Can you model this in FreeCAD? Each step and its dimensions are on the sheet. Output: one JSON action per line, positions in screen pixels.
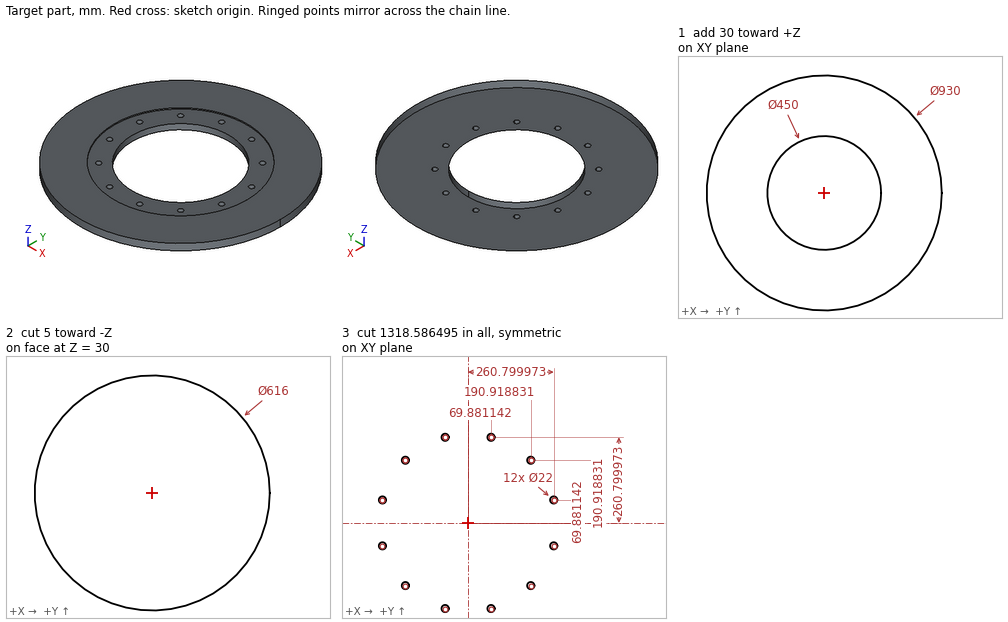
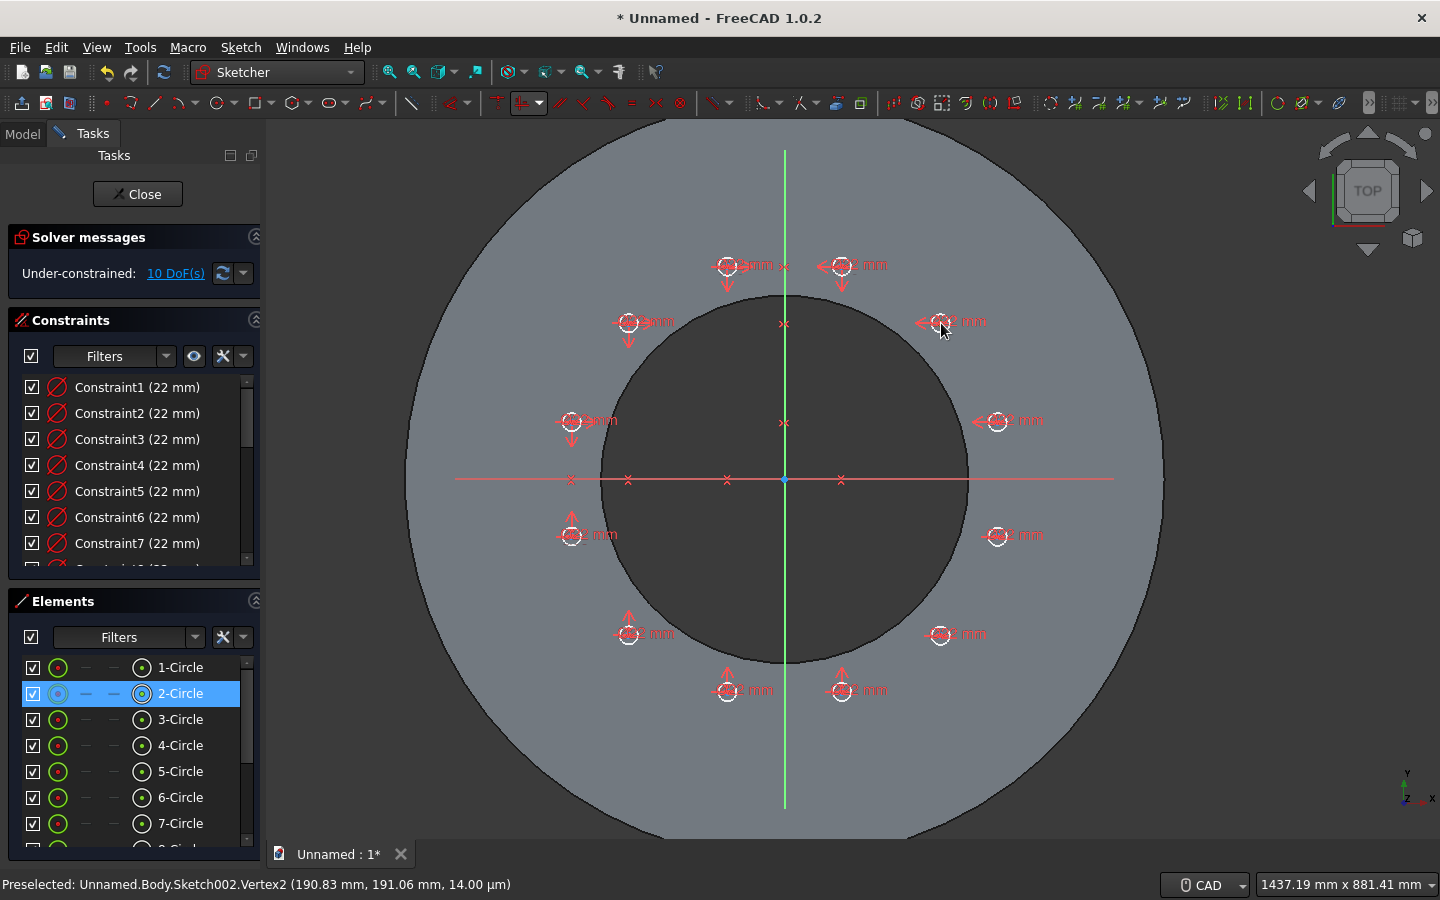
{"action": "left_click", "coordinate": [941, 636]}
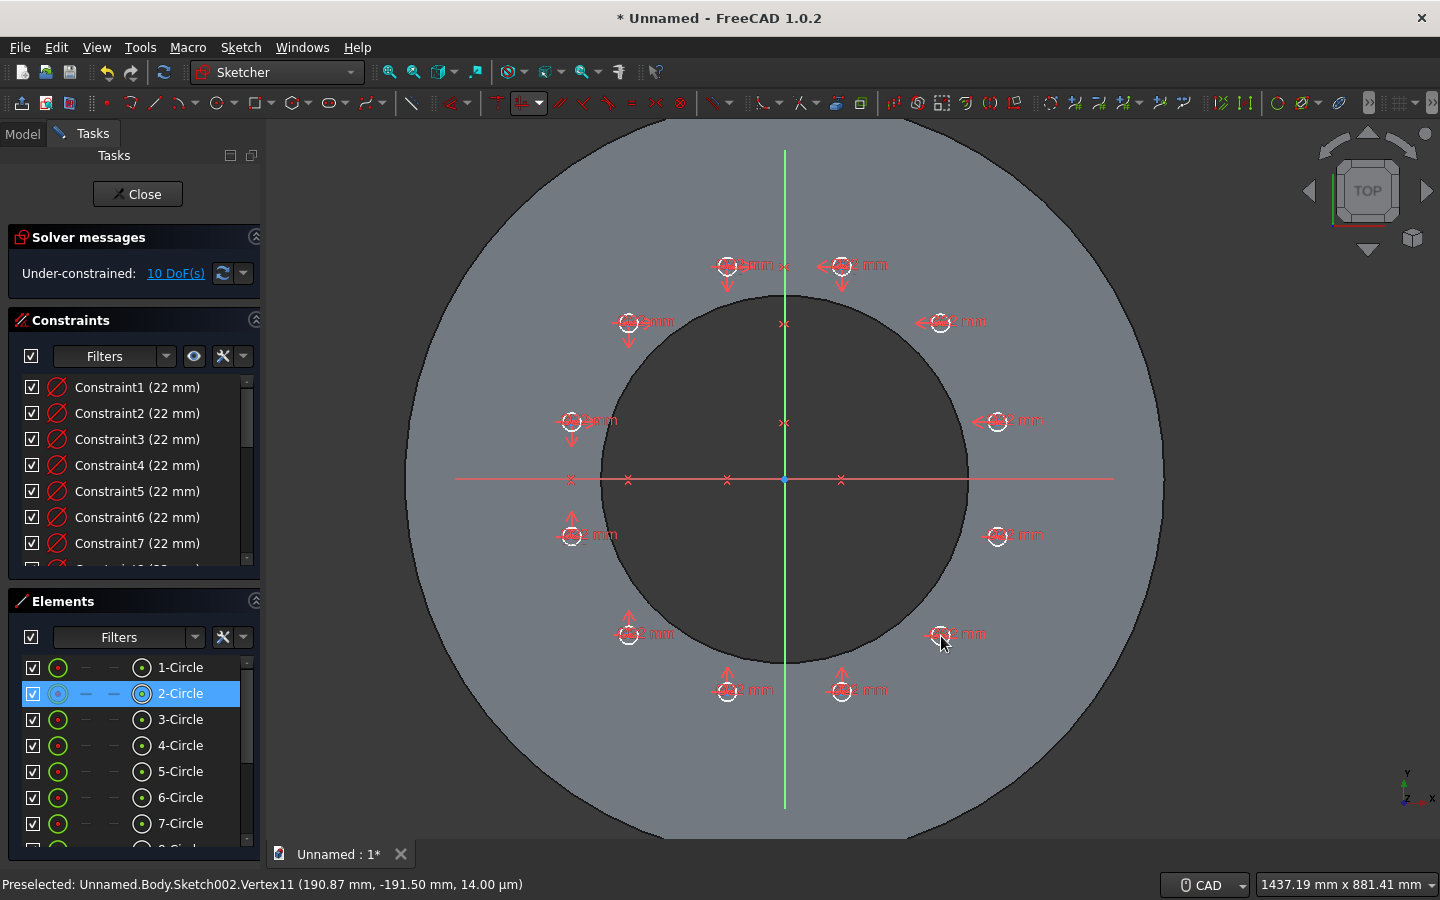
{"action": "left_click", "coordinate": [504, 479]}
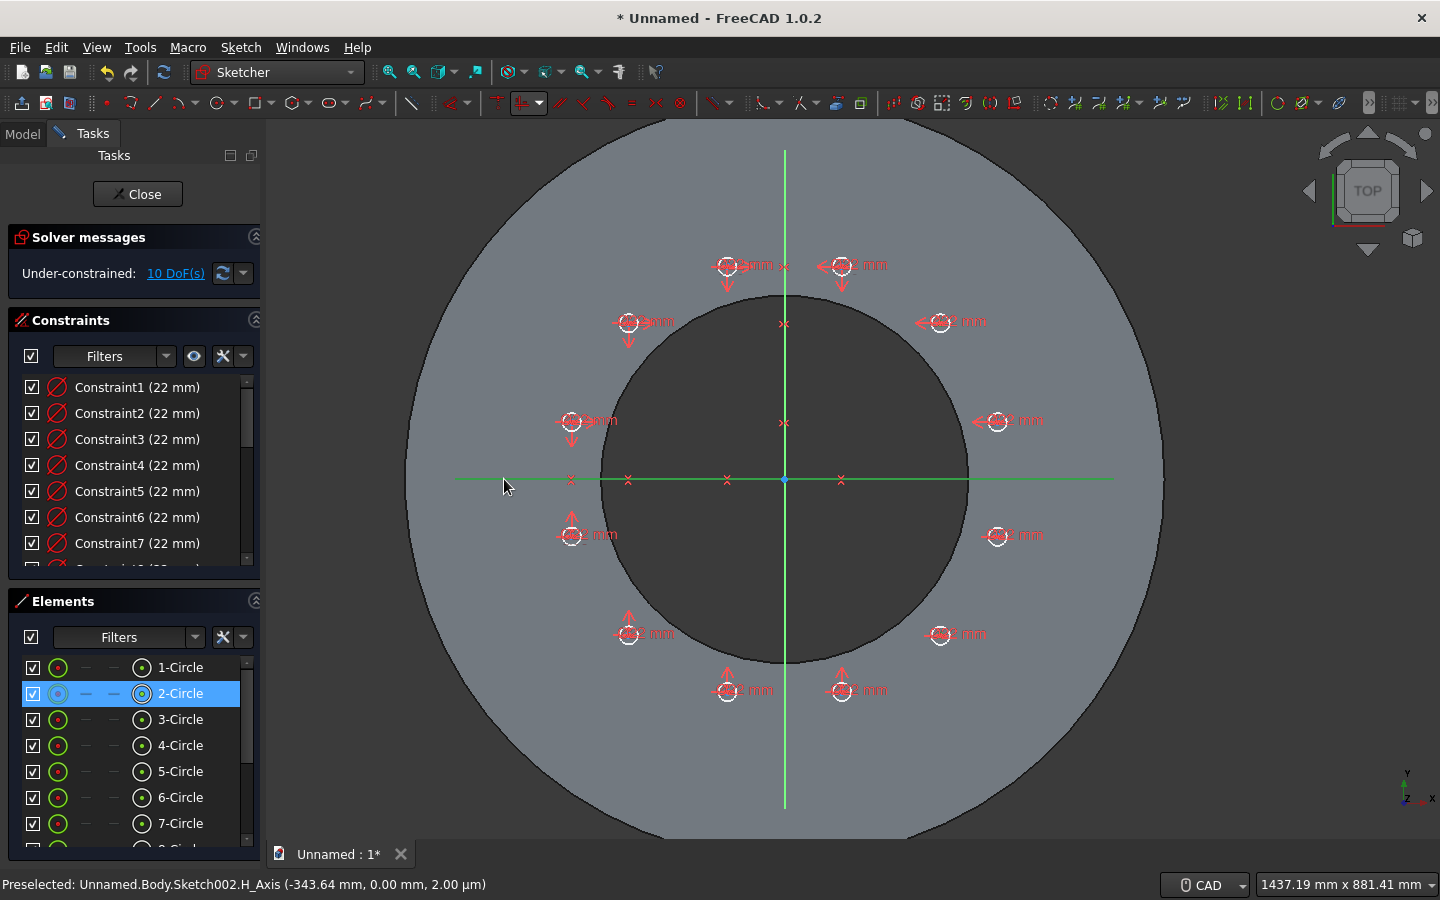
{"action": "left_click", "coordinate": [656, 104]}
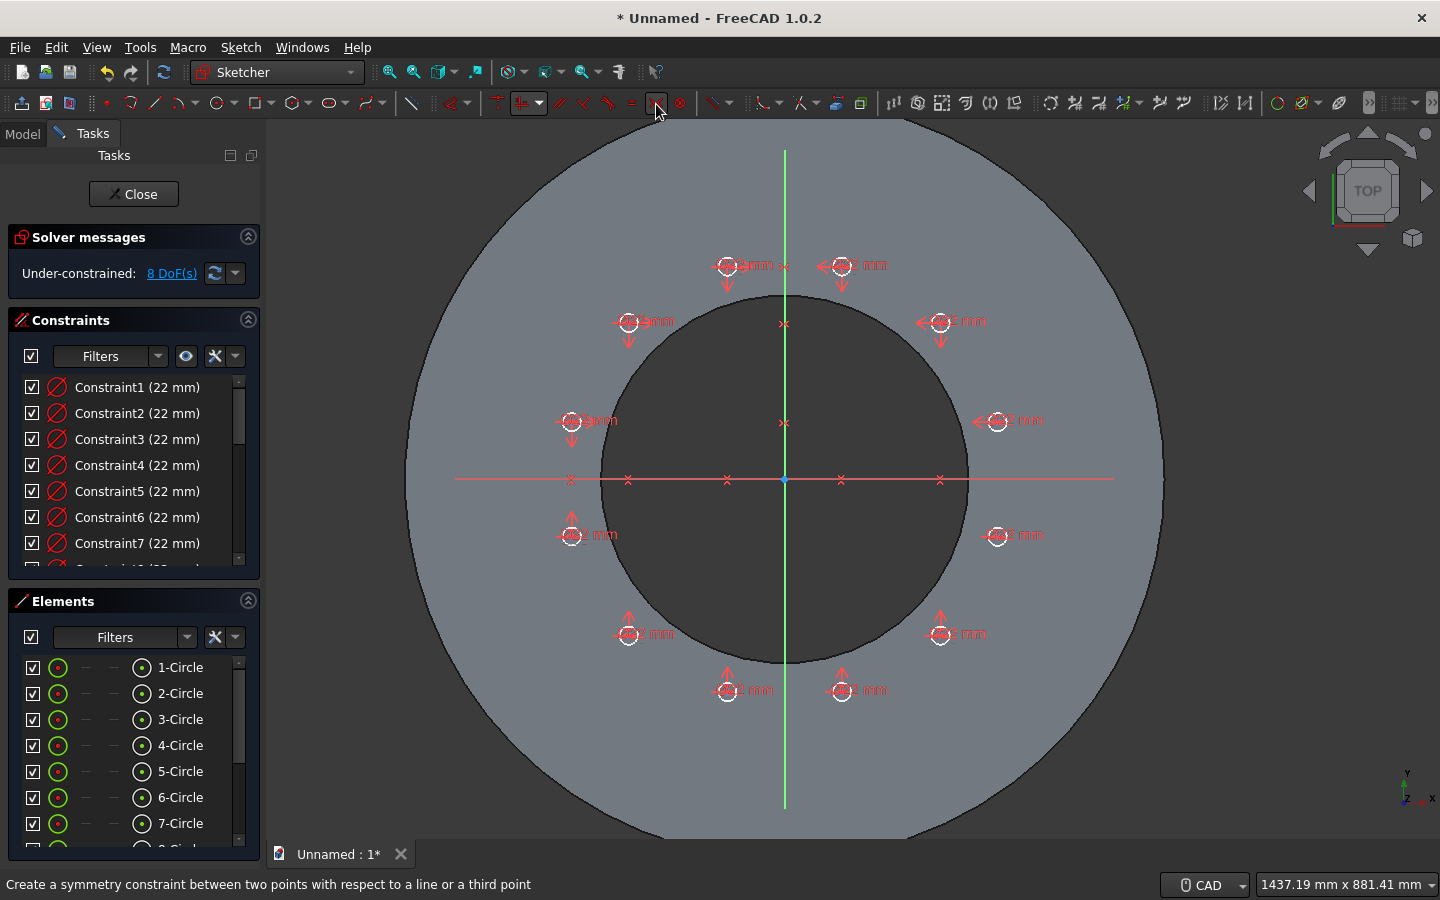
{"action": "left_click", "coordinate": [998, 422]}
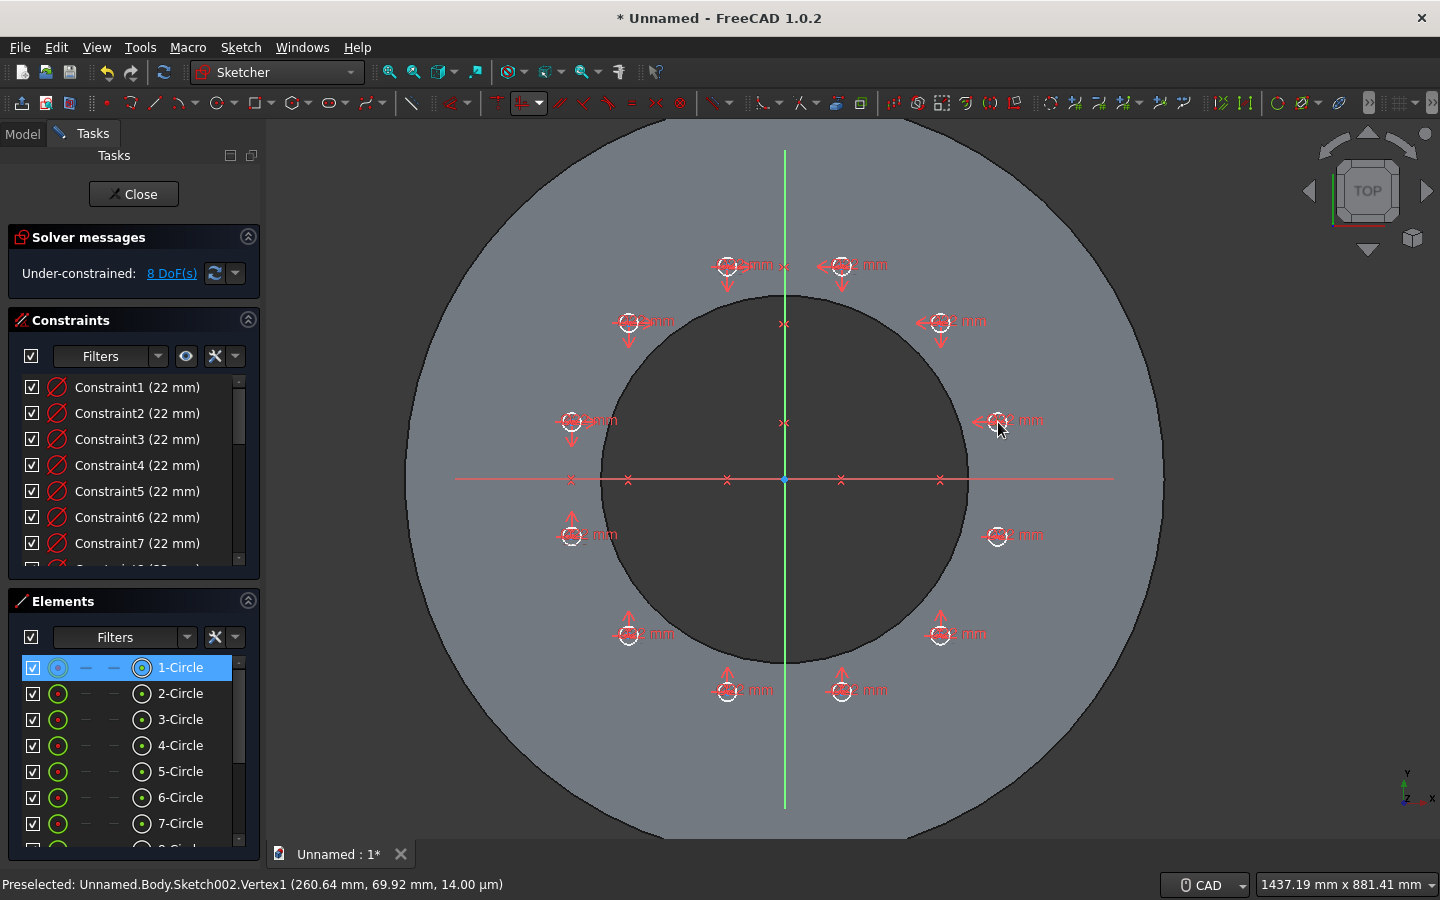
{"action": "left_click", "coordinate": [998, 537]}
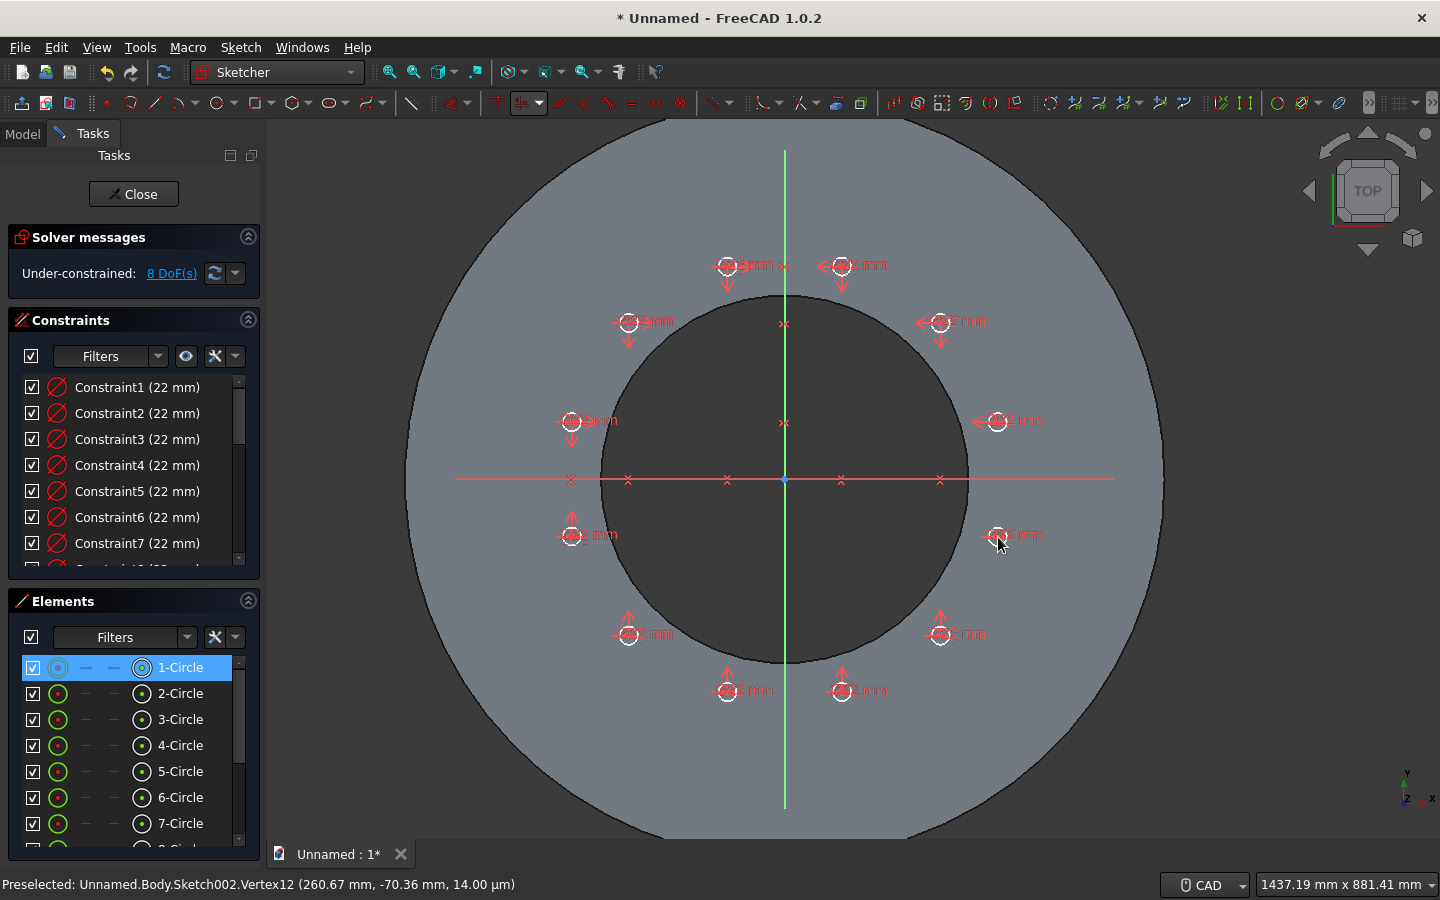
{"action": "left_click", "coordinate": [504, 479]}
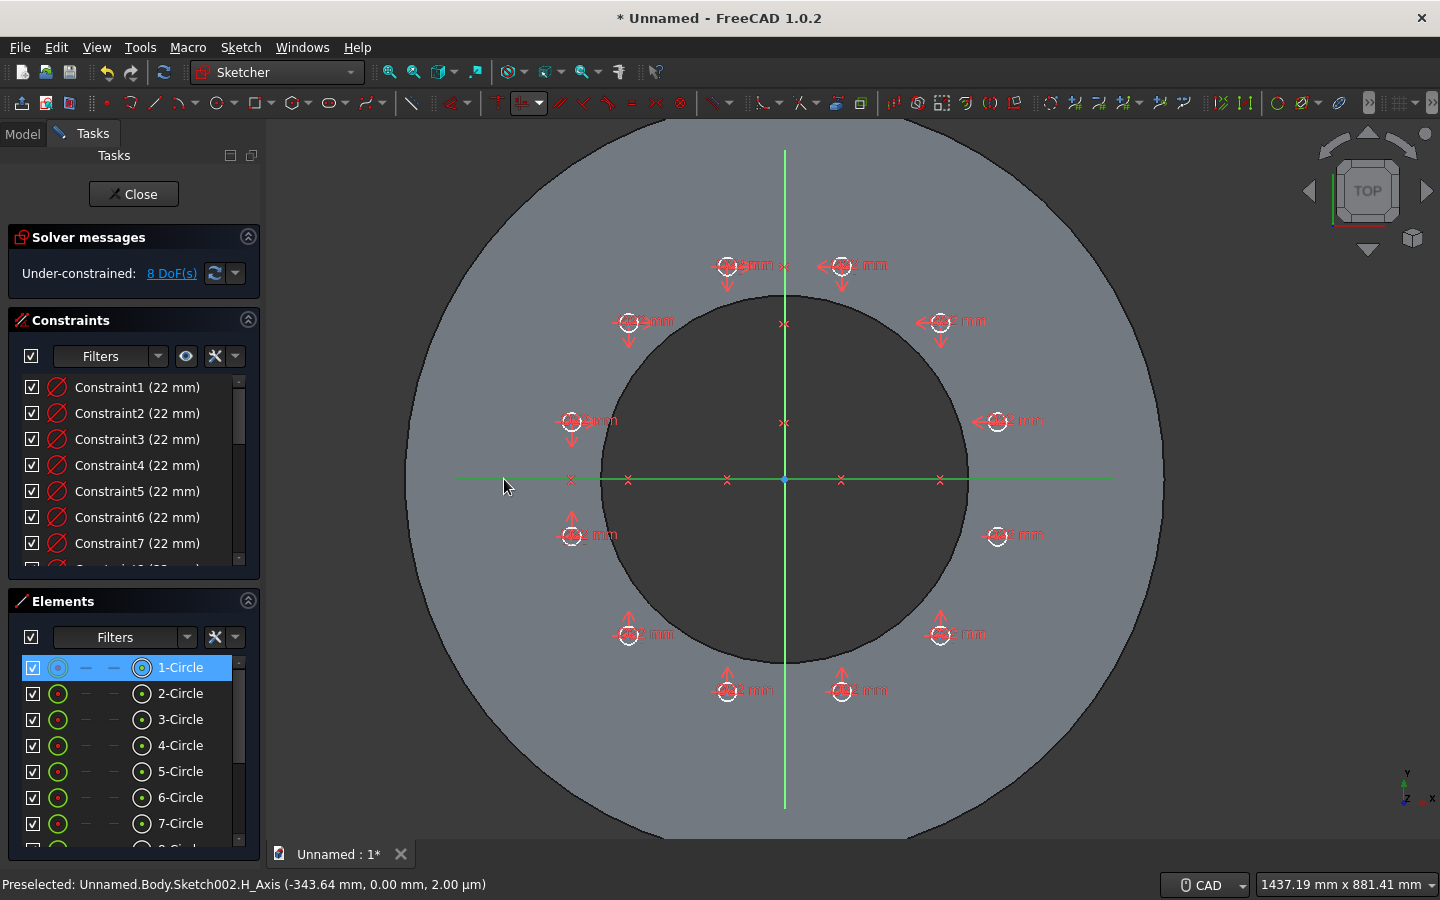
{"action": "left_click", "coordinate": [656, 104]}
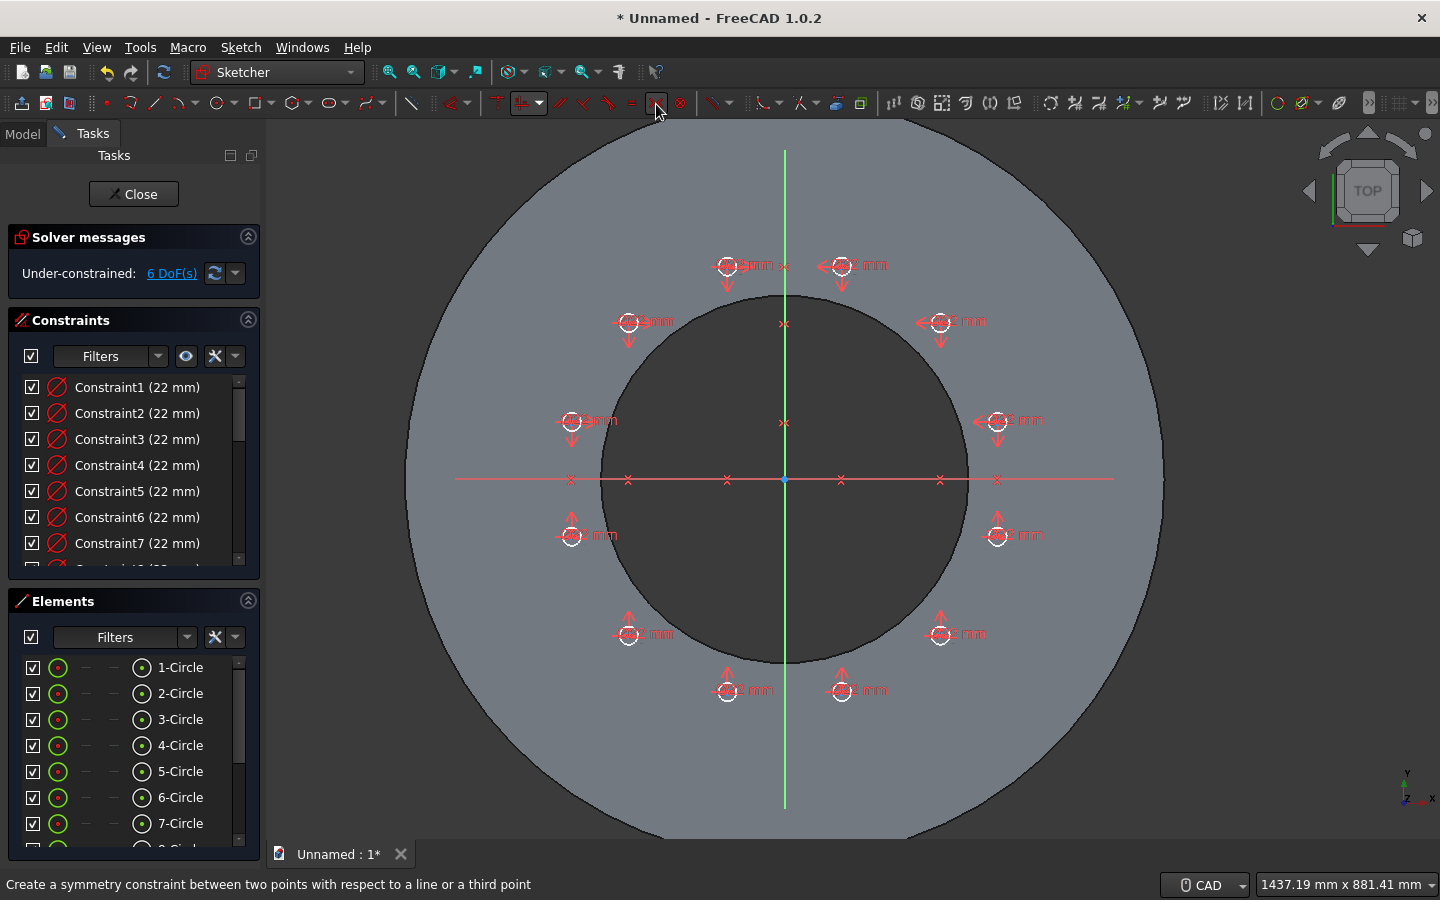
{"action": "left_click", "coordinate": [450, 104]}